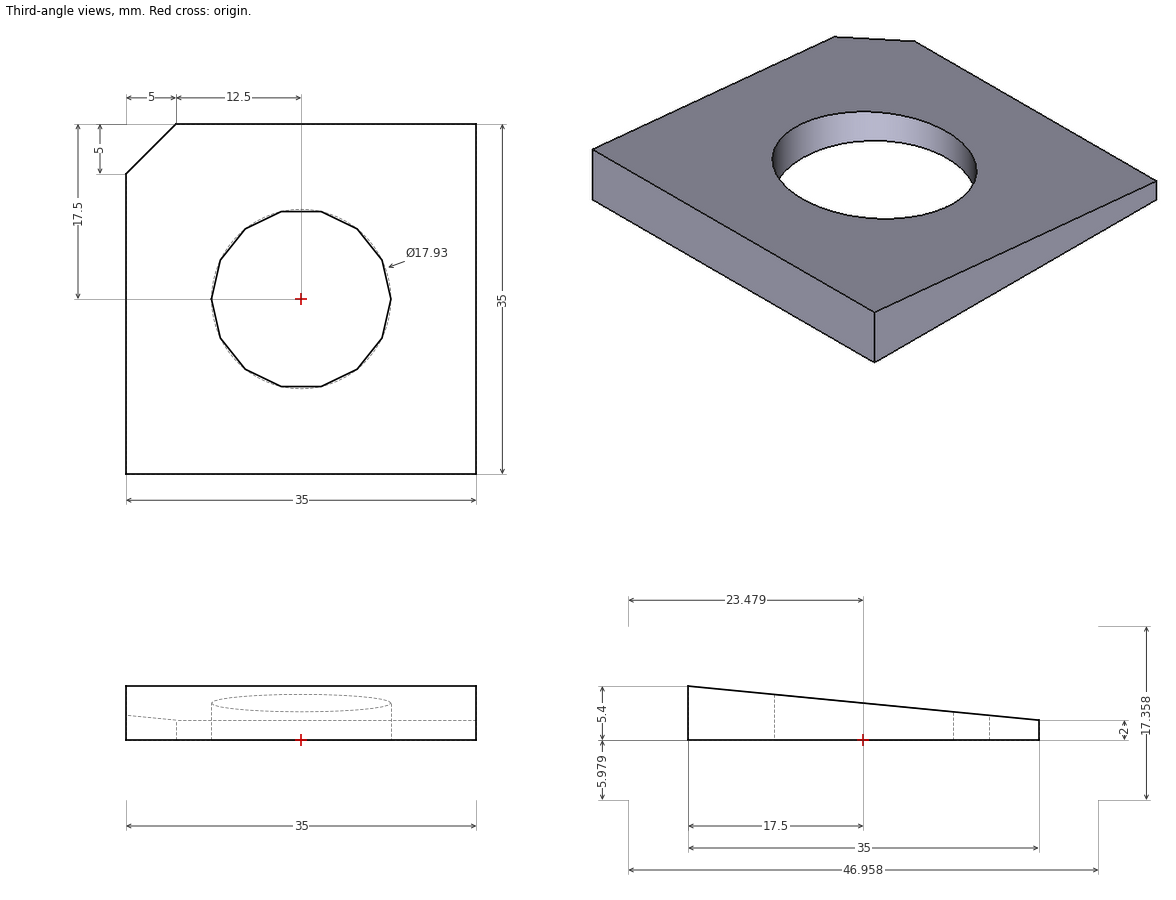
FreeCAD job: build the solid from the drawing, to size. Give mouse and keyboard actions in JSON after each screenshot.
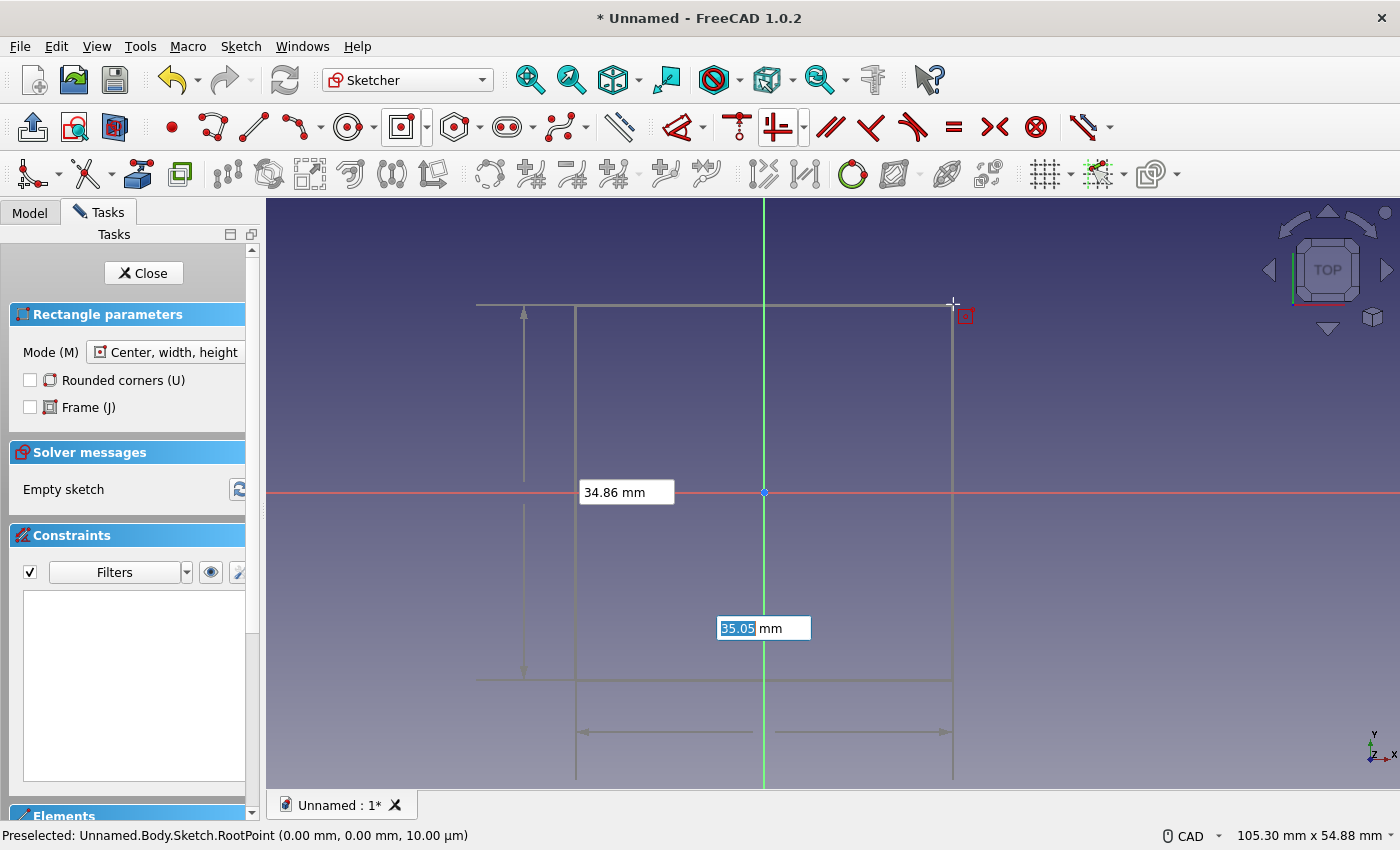
{"action": "type", "text": "35"}
{"action": "key", "text": "Tab"}
{"action": "type", "text": "35"}
{"action": "key", "text": "Return"}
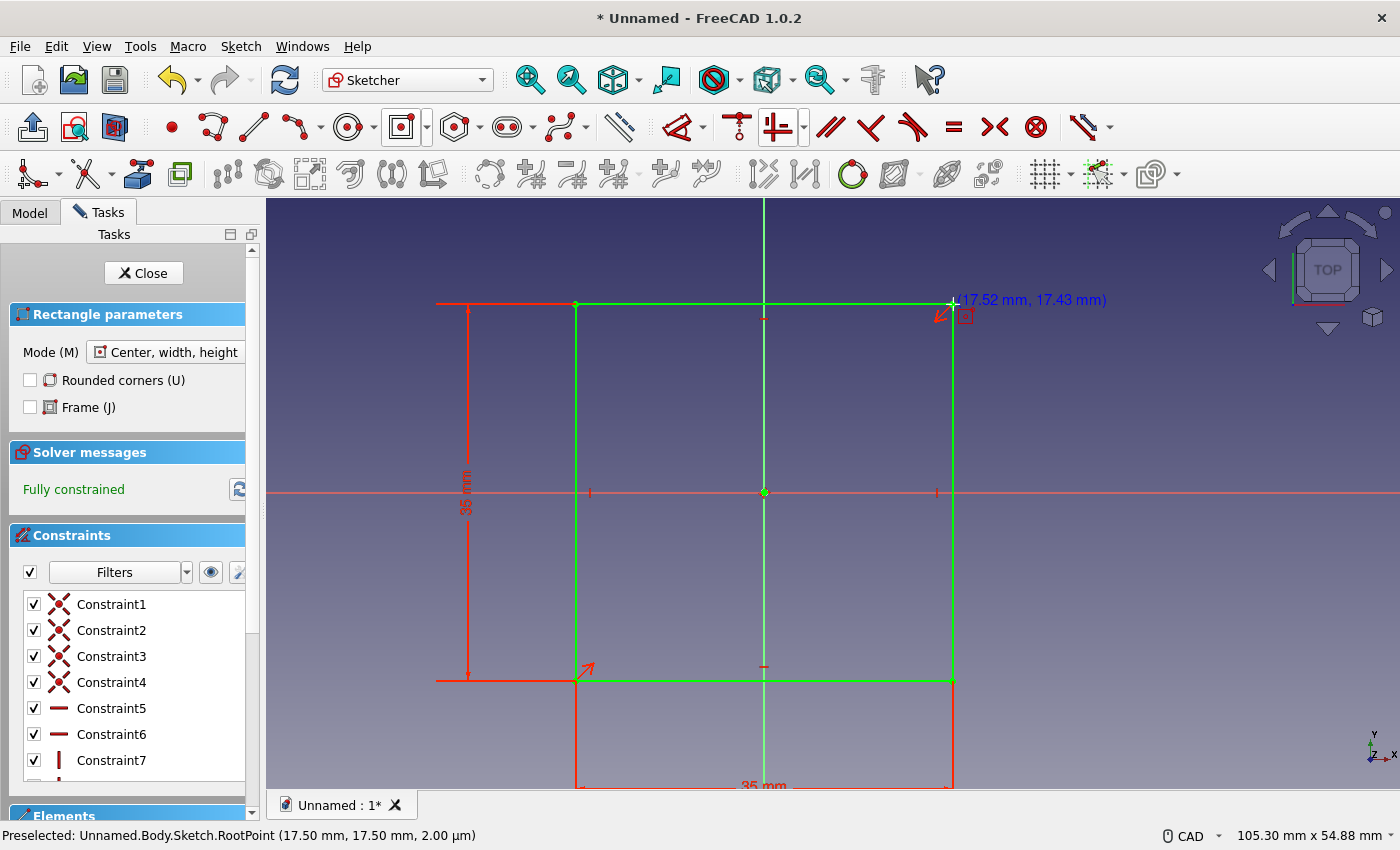
{"action": "key", "text": "g c"}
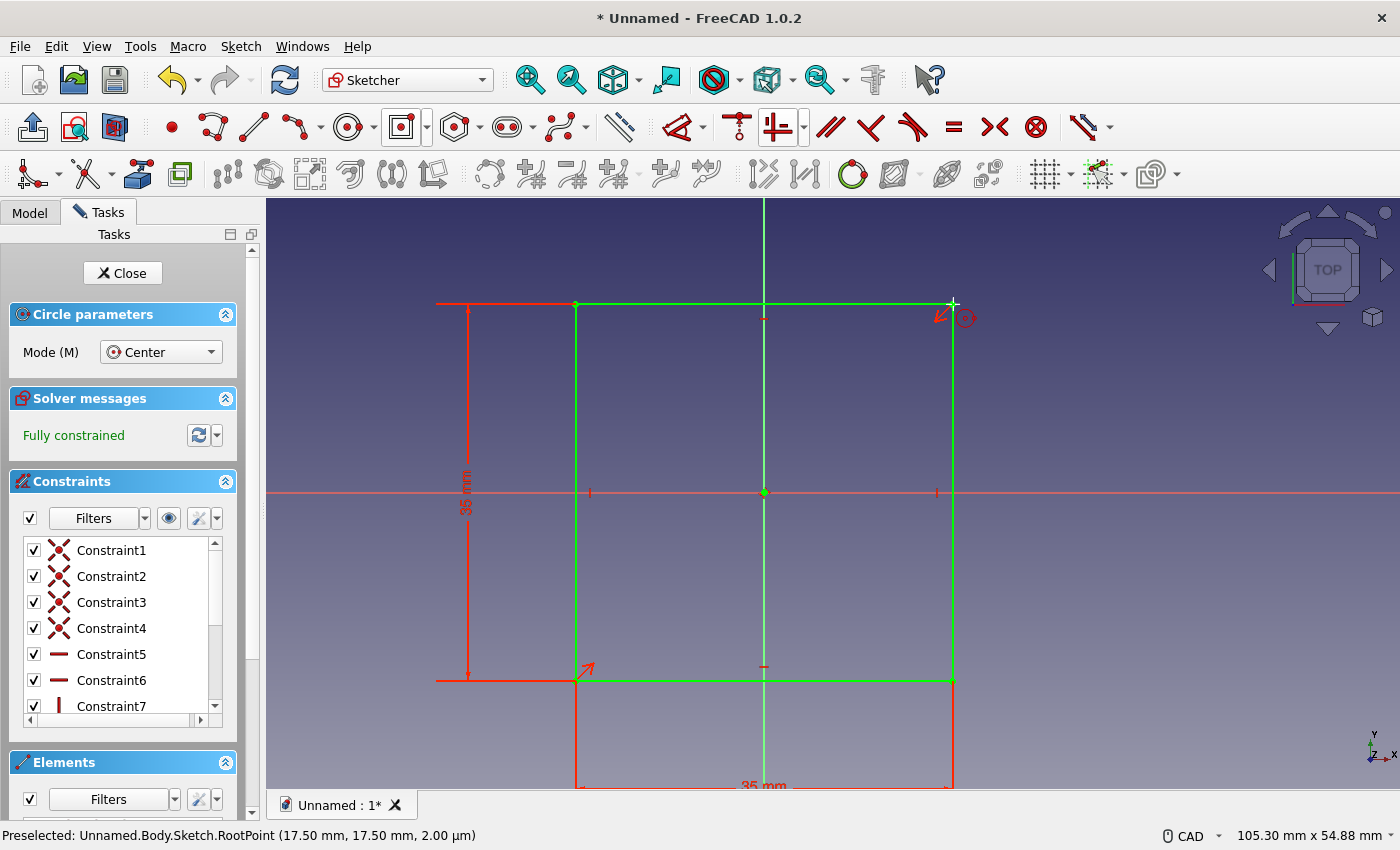
{"action": "left_click", "coordinate": [764, 493]}
{"action": "mouse_move", "coordinate": [833, 424]}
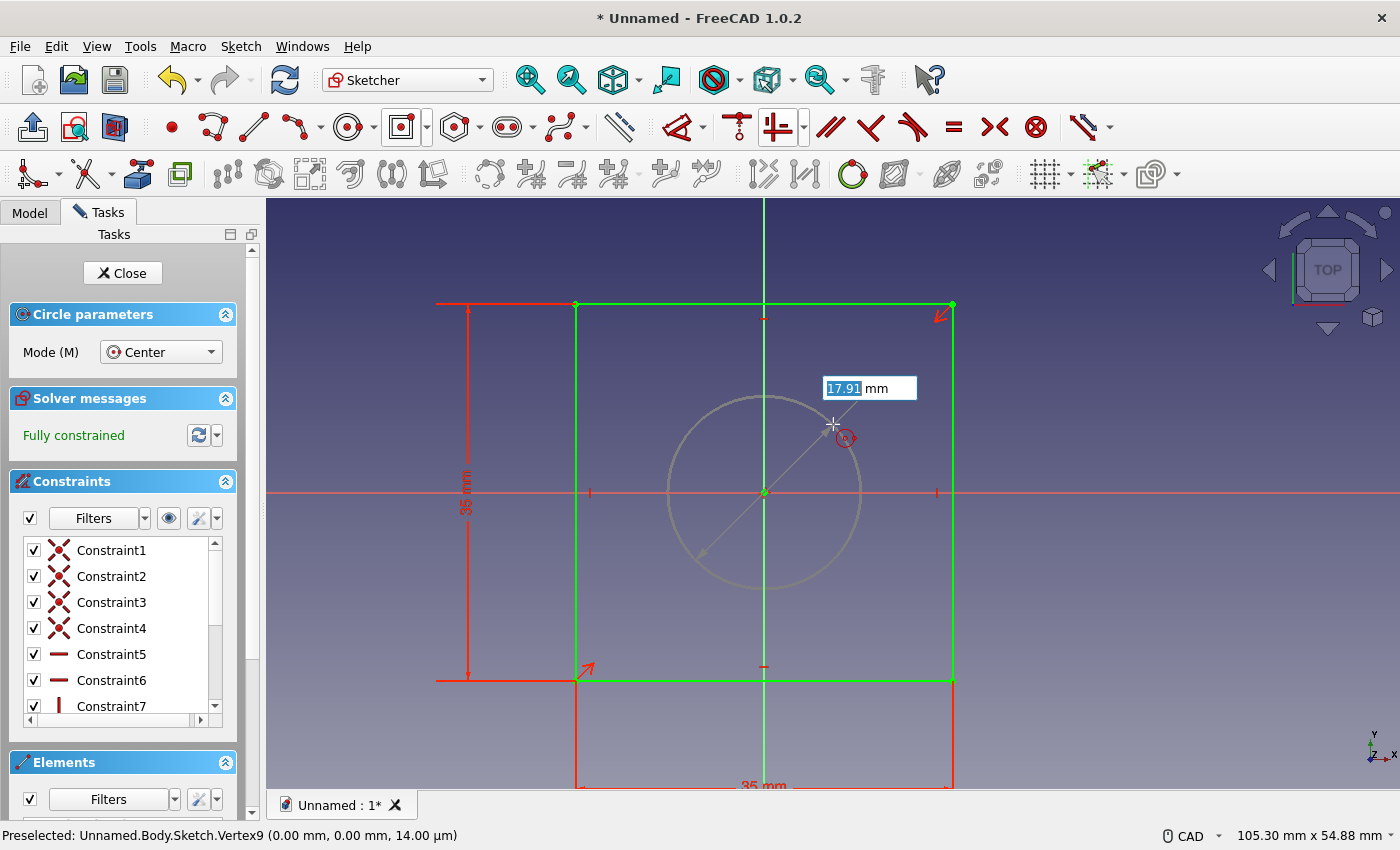
{"action": "type", "text": "17.93"}
{"action": "key", "text": "Return"}
{"action": "key", "text": "Escape"}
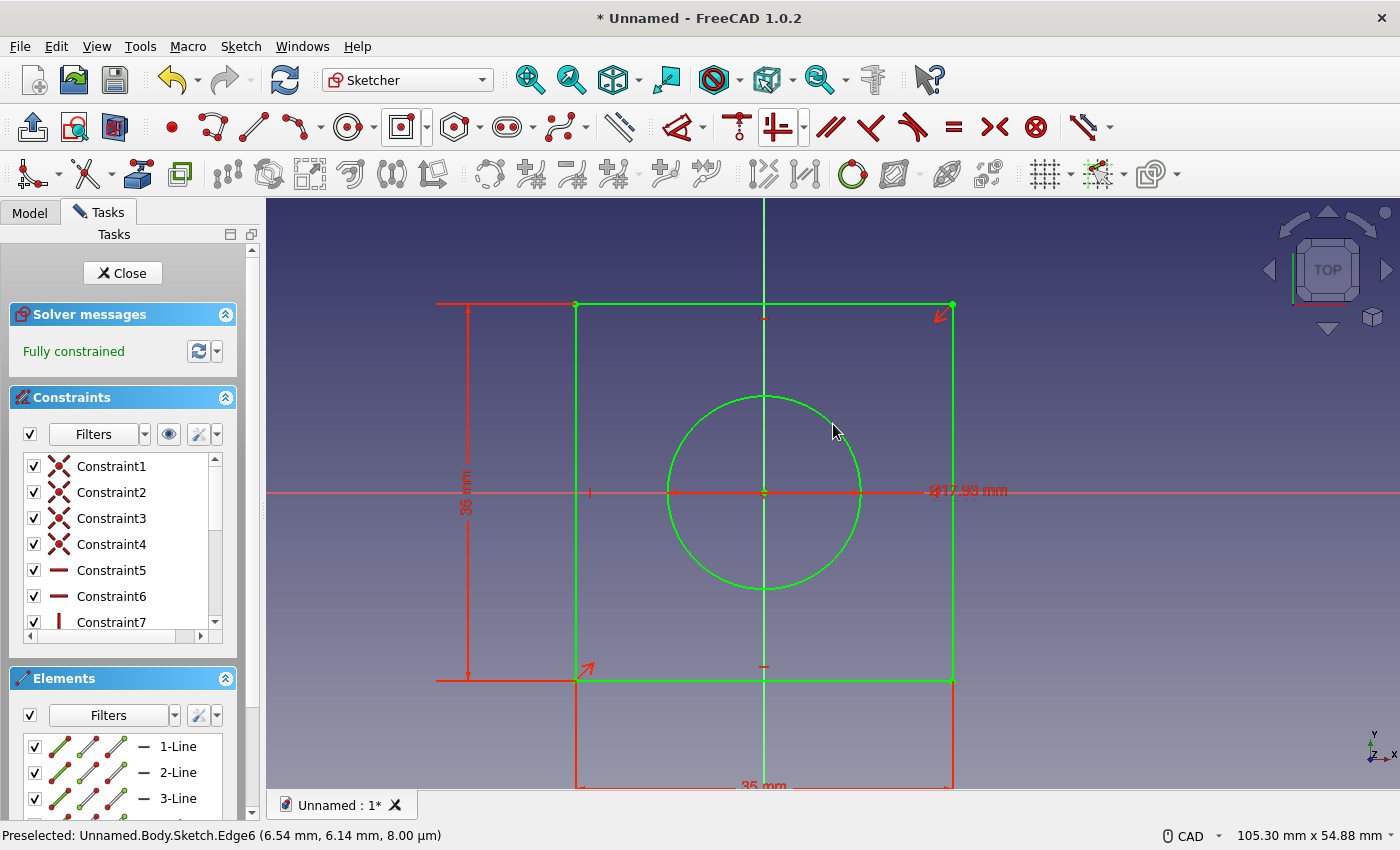
{"action": "left_click", "coordinate": [123, 273]}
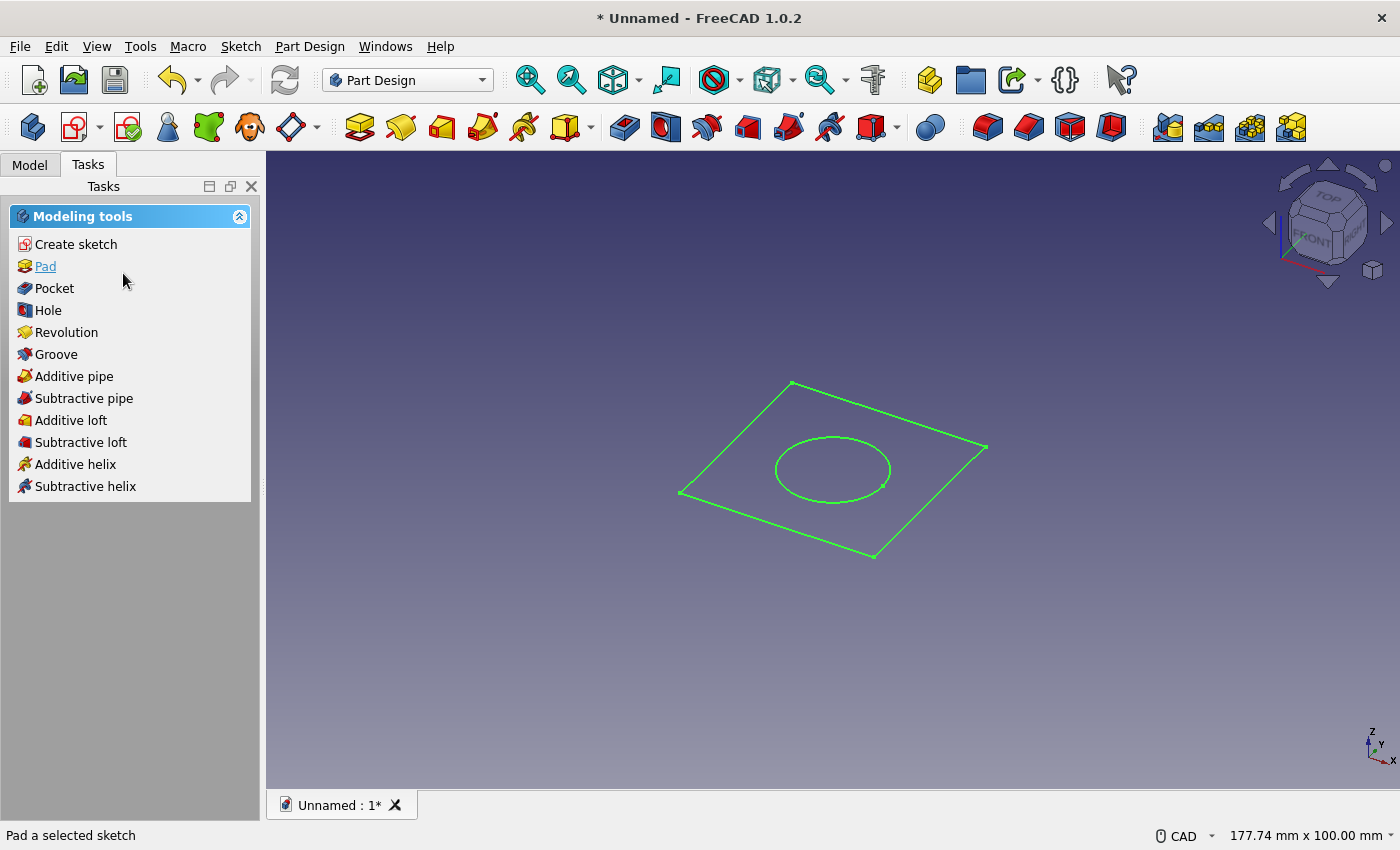
{"action": "left_click", "coordinate": [360, 128]}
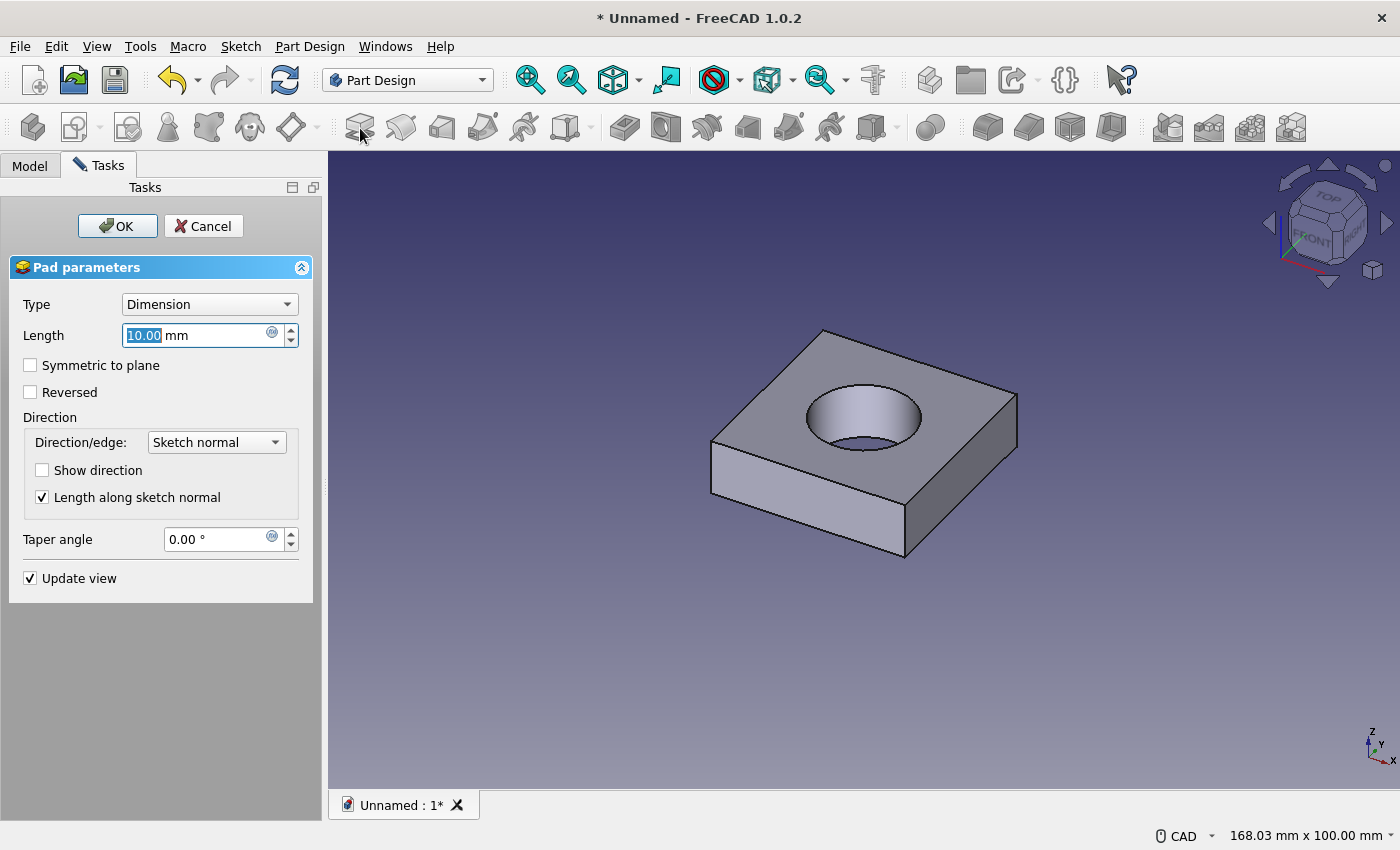
{"action": "type", "text": "5.4"}
{"action": "key", "text": "Tab"}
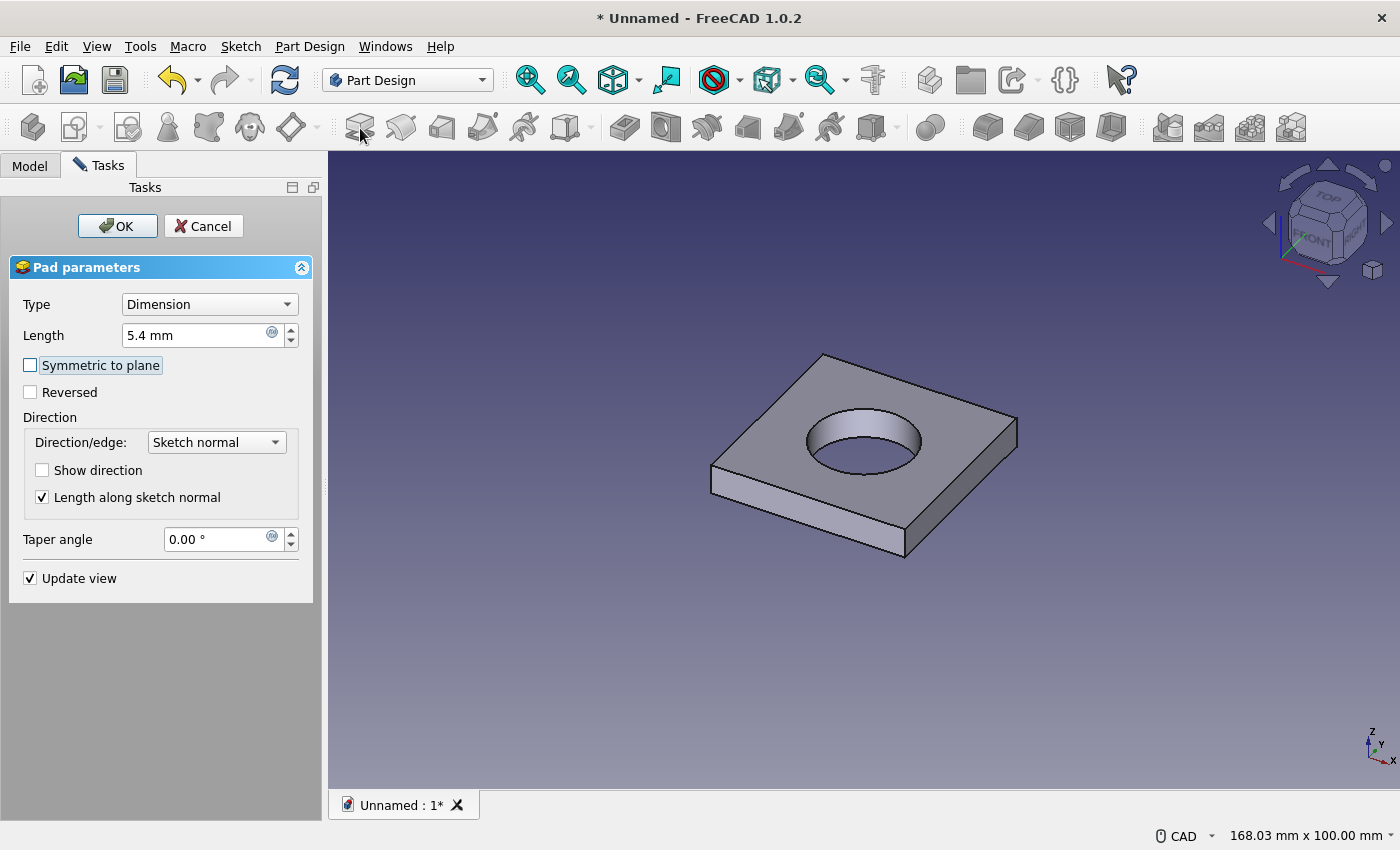
{"action": "left_click", "coordinate": [118, 226]}